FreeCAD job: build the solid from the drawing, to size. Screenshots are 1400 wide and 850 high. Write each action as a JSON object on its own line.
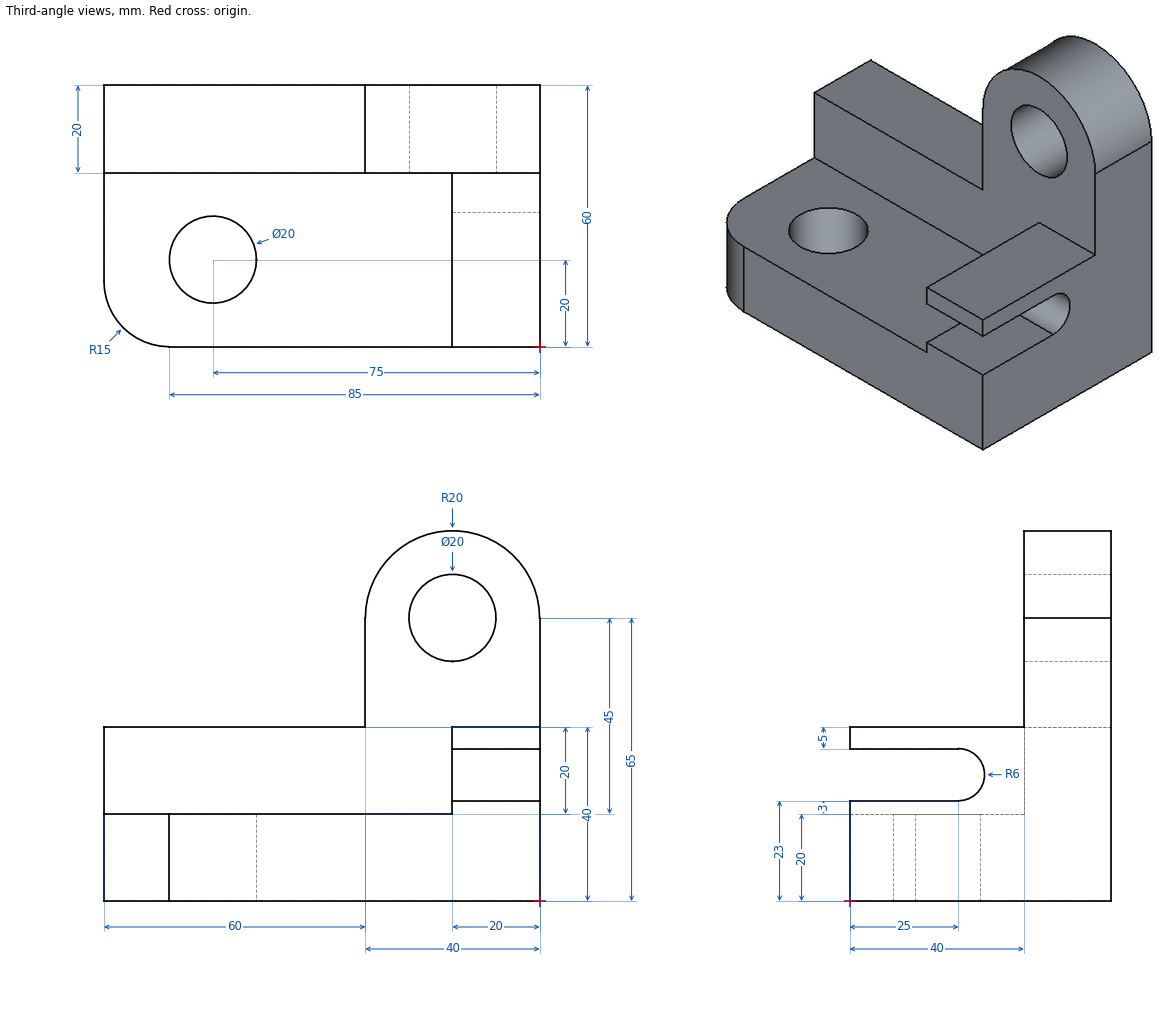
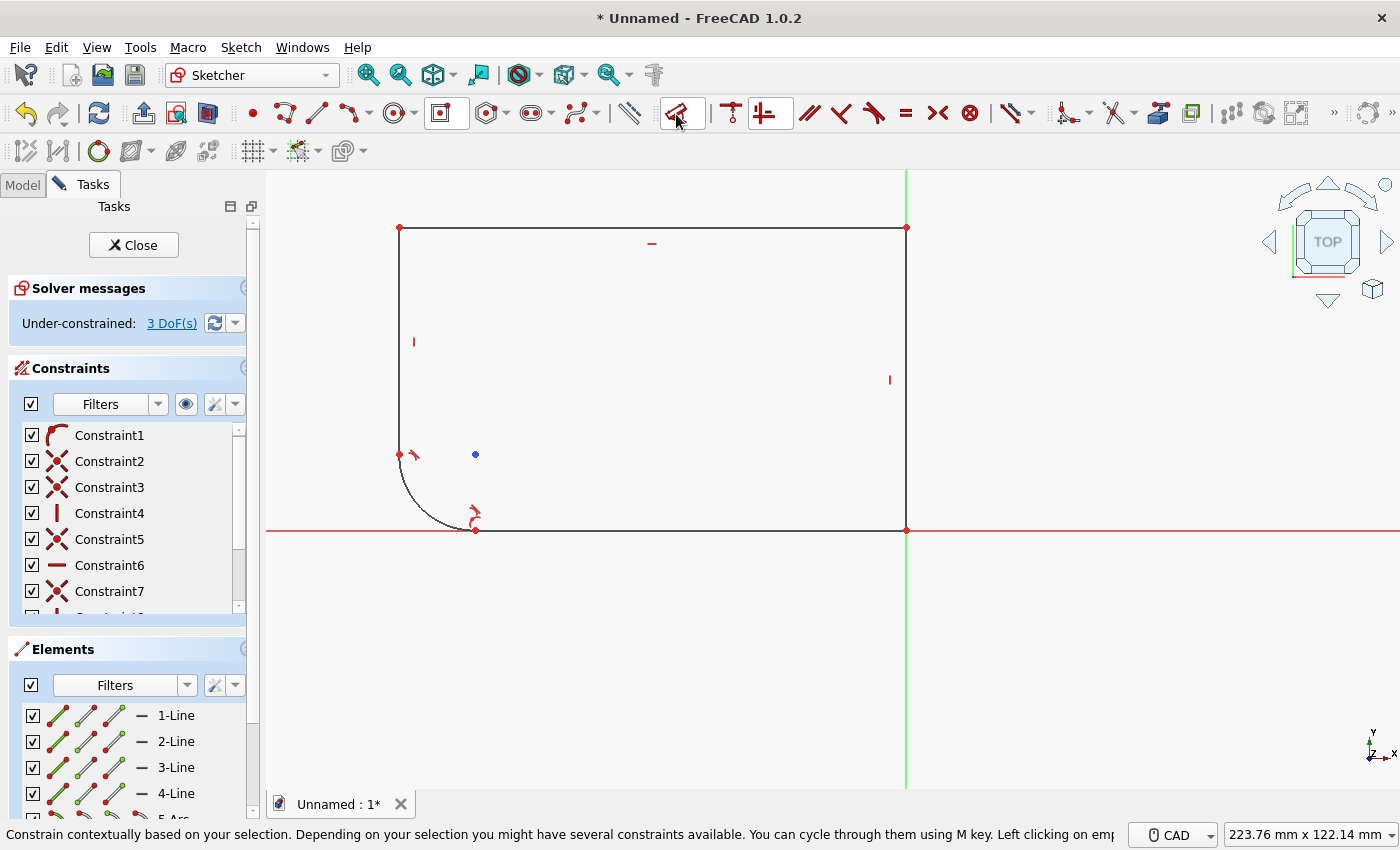
{"action": "left_click", "coordinate": [407, 489]}
{"action": "left_click", "coordinate": [378, 503]}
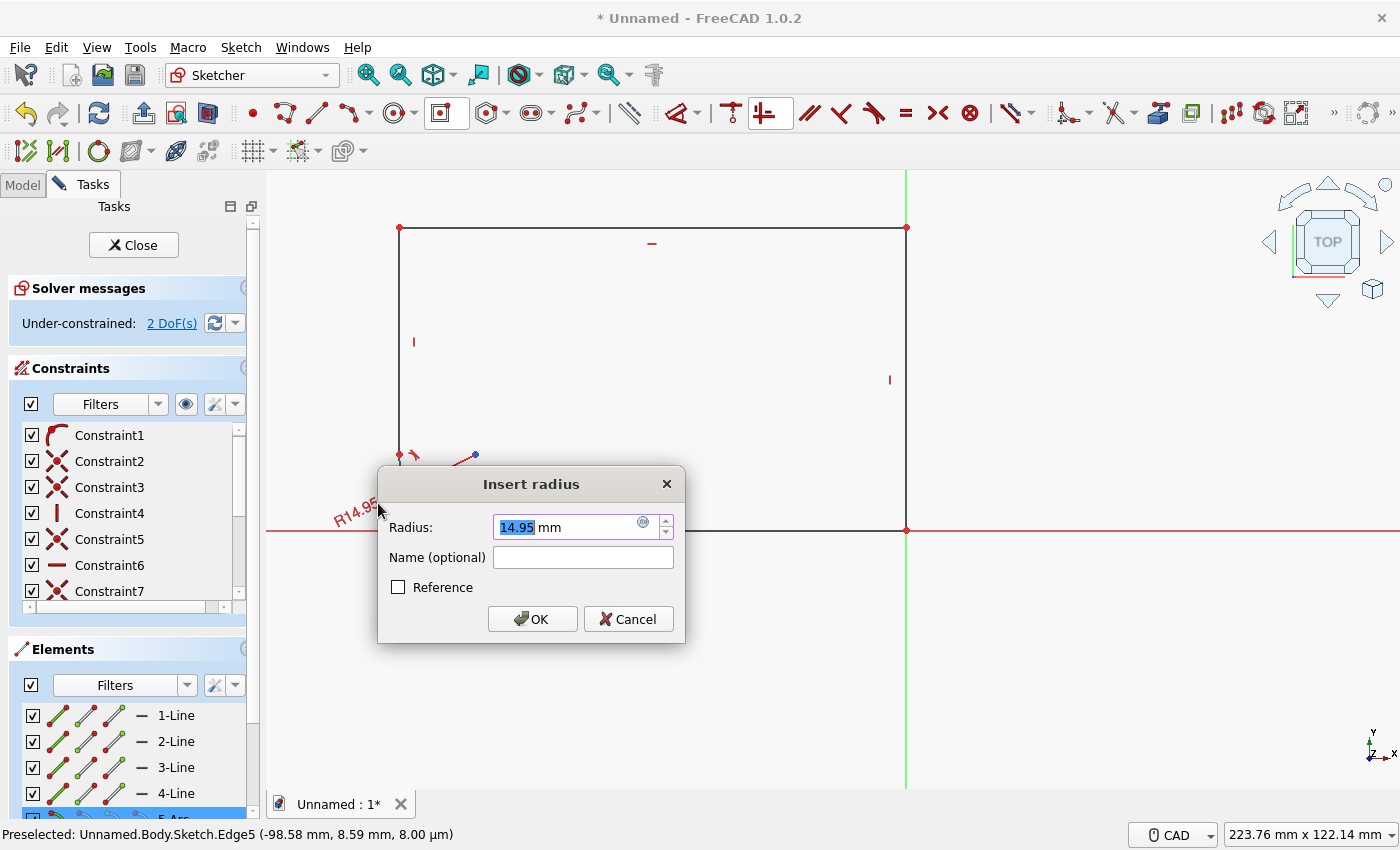
{"action": "type", "text": "15"}
{"action": "key", "text": "Return"}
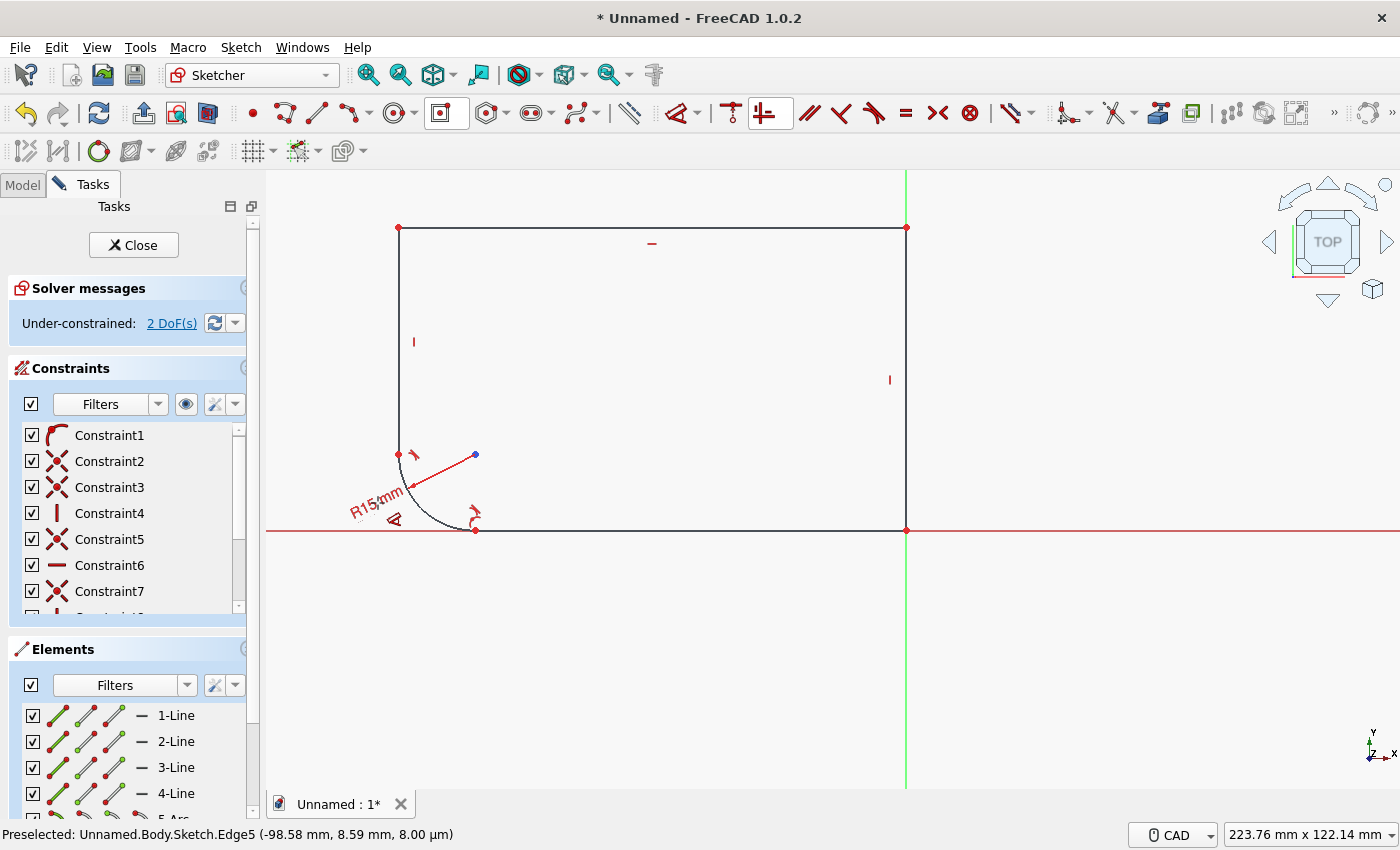
{"action": "left_click", "coordinate": [604, 531]}
{"action": "left_click", "coordinate": [691, 565]}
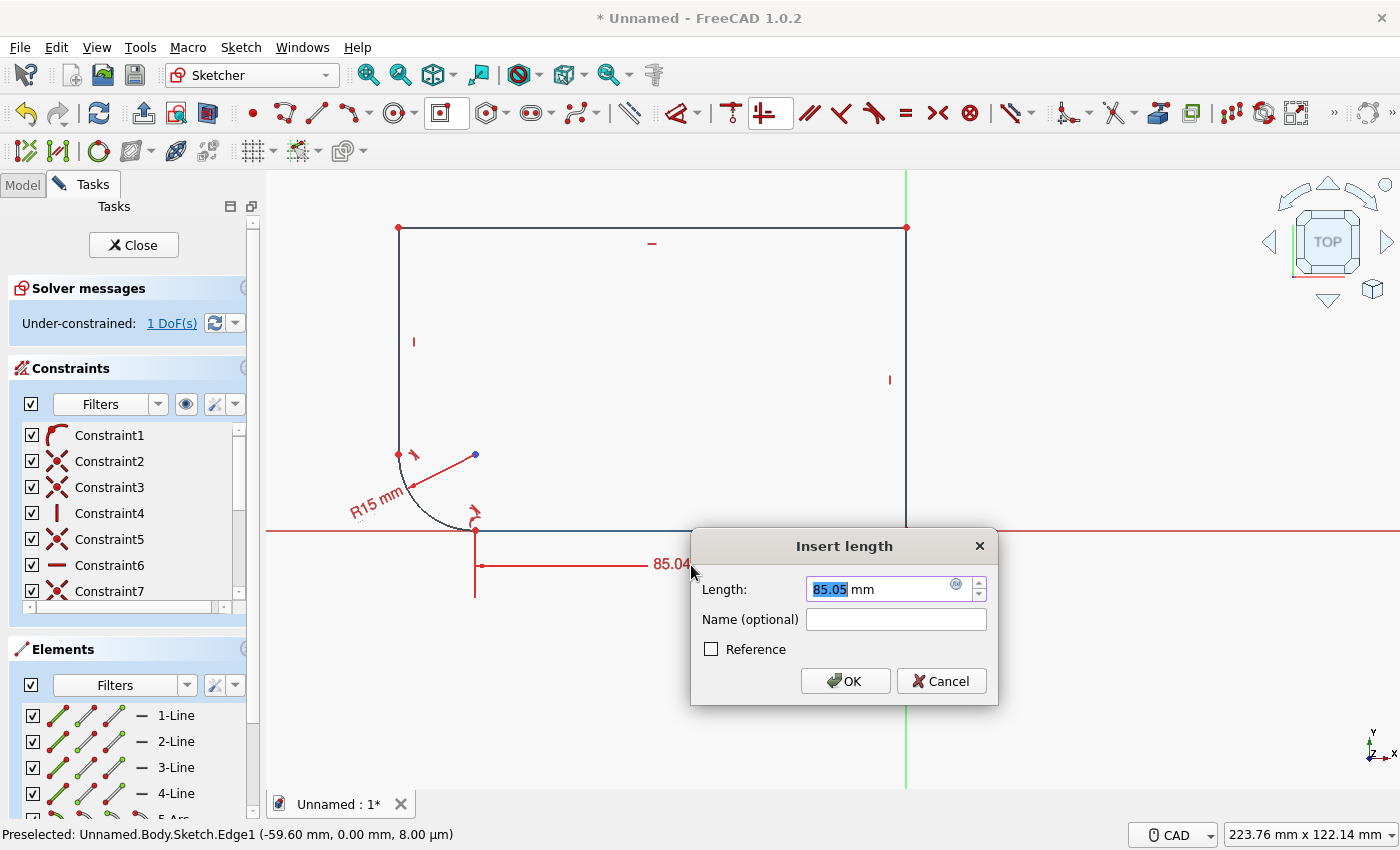
{"action": "type", "text": "85"}
{"action": "key", "text": "Return"}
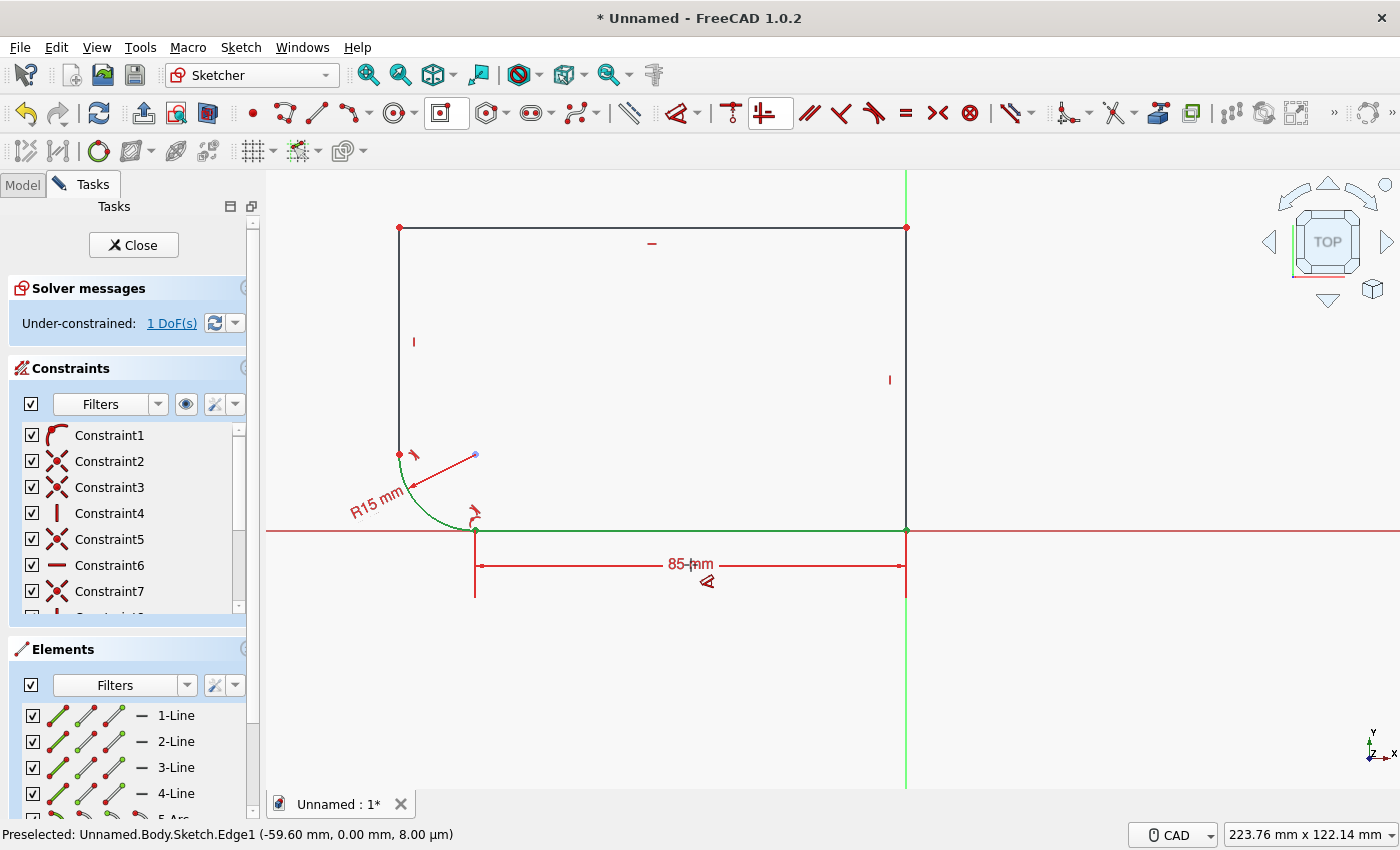
{"action": "left_click", "coordinate": [906, 440]}
{"action": "left_click", "coordinate": [940, 379]}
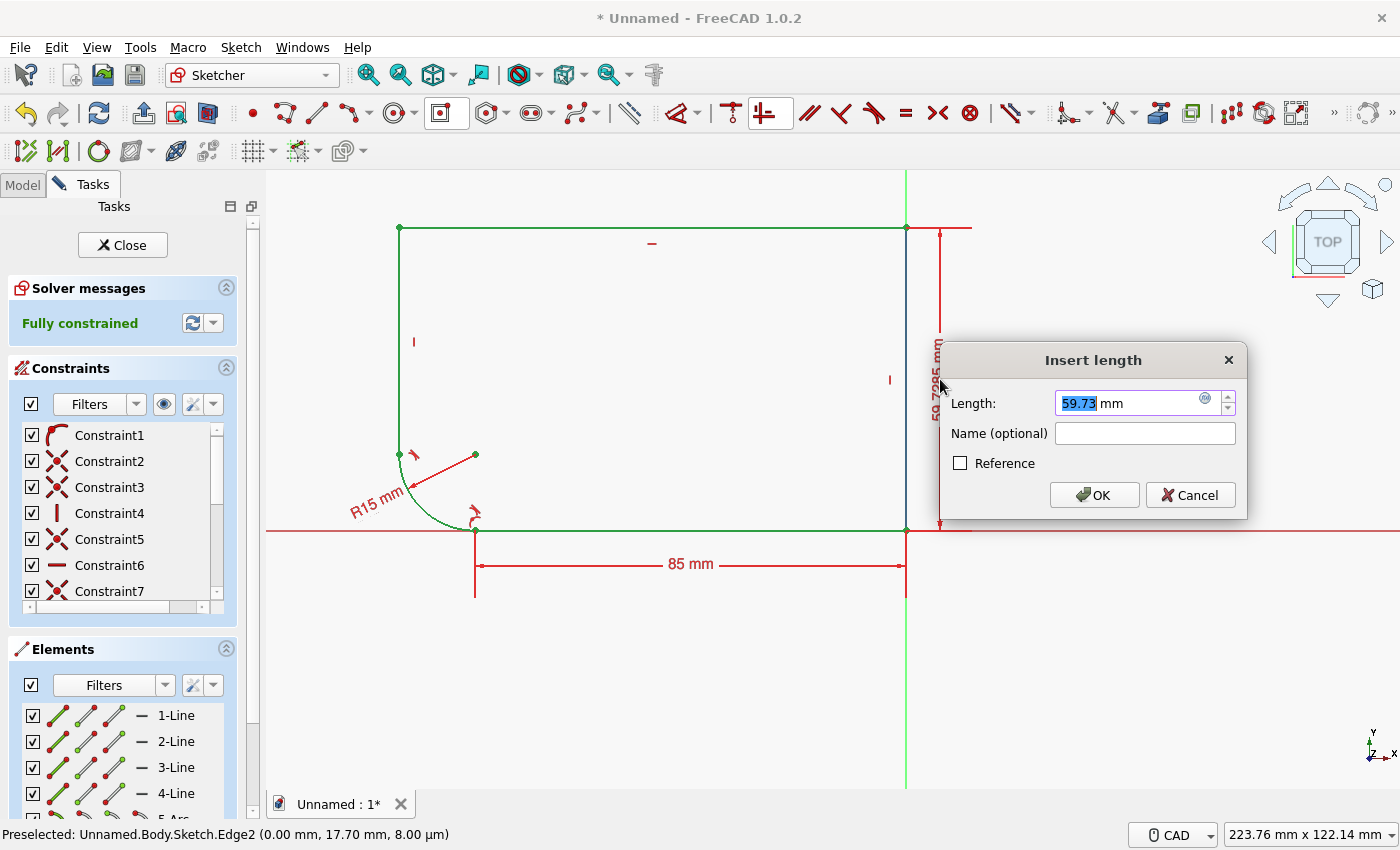
{"action": "type", "text": "60"}
{"action": "key", "text": "Return"}
{"action": "key", "text": "Escape"}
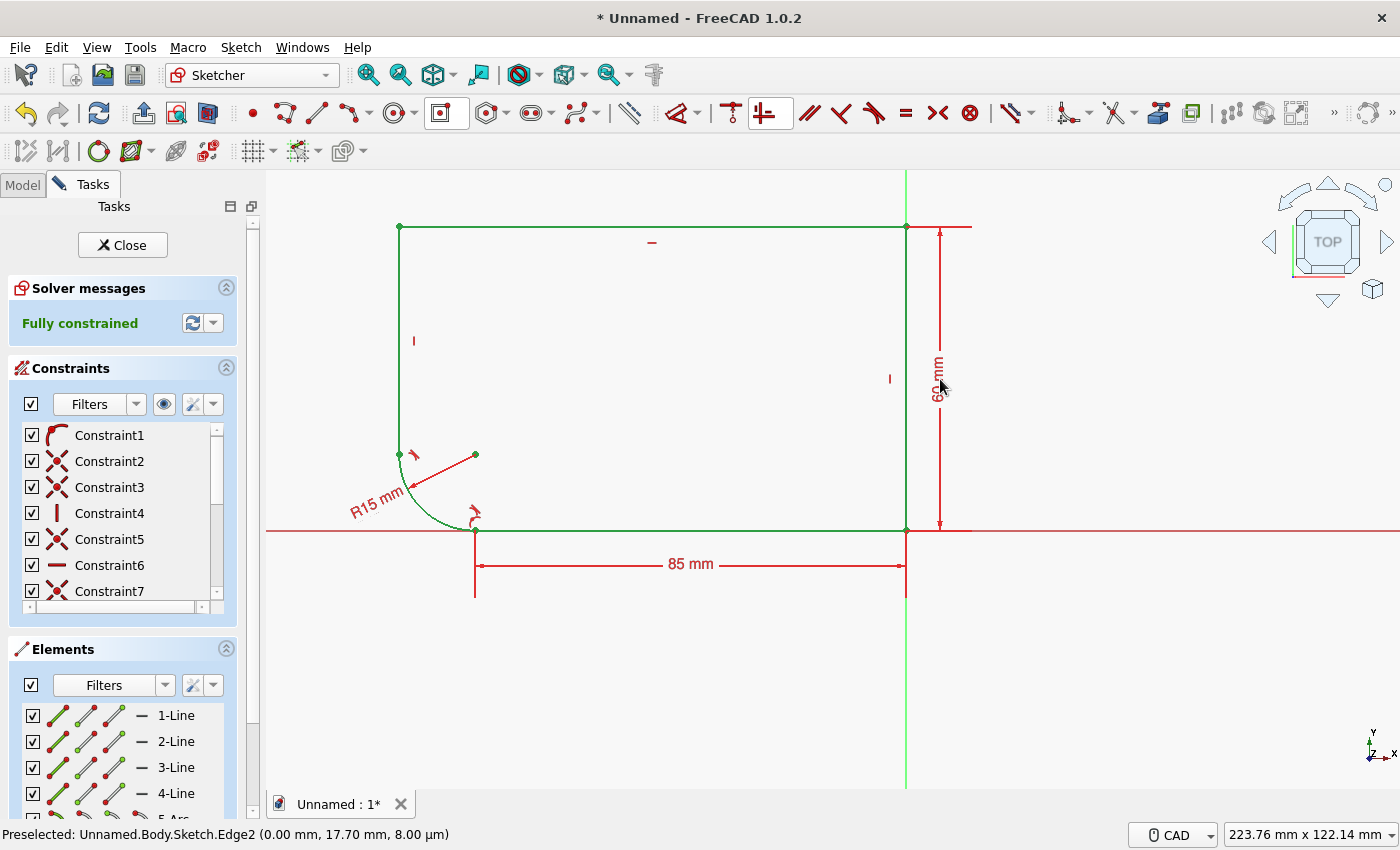
{"action": "left_click", "coordinate": [123, 245]}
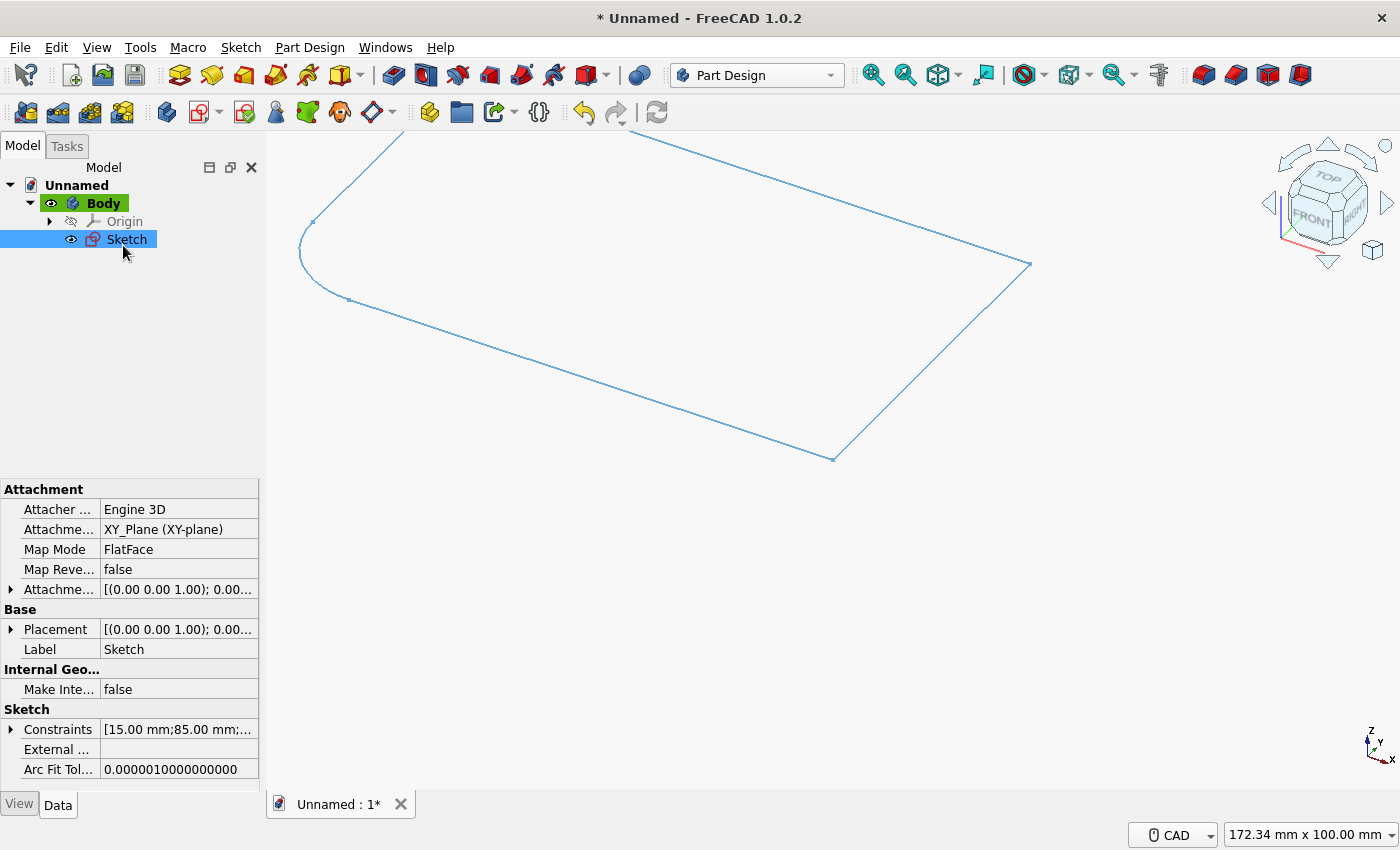
{"action": "left_click", "coordinate": [180, 76]}